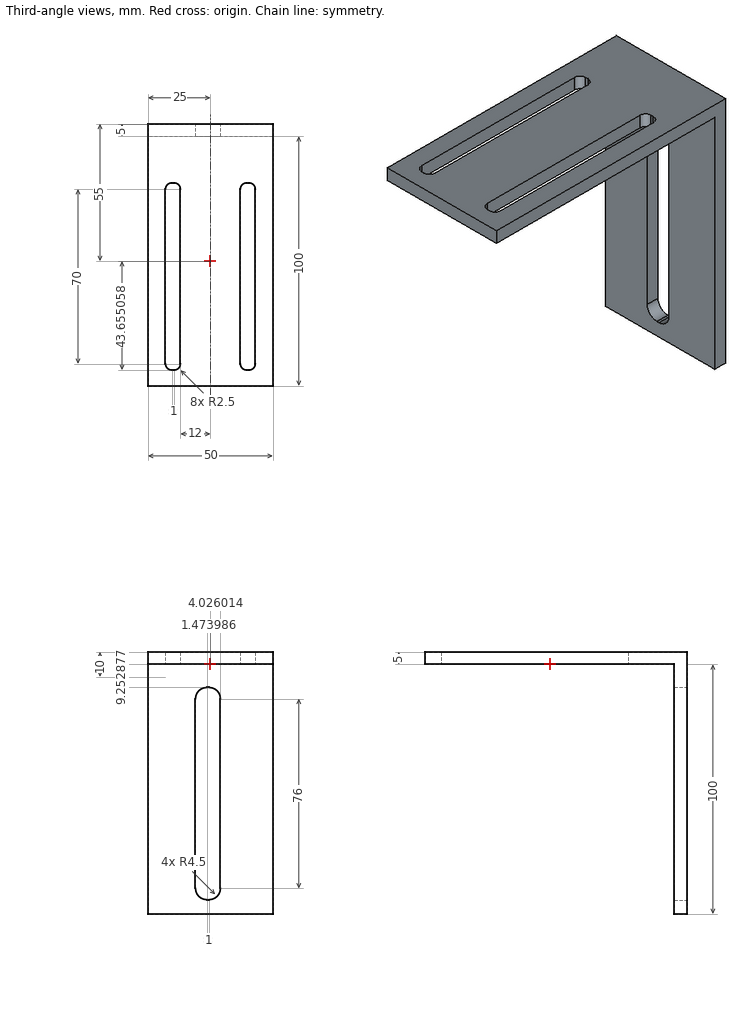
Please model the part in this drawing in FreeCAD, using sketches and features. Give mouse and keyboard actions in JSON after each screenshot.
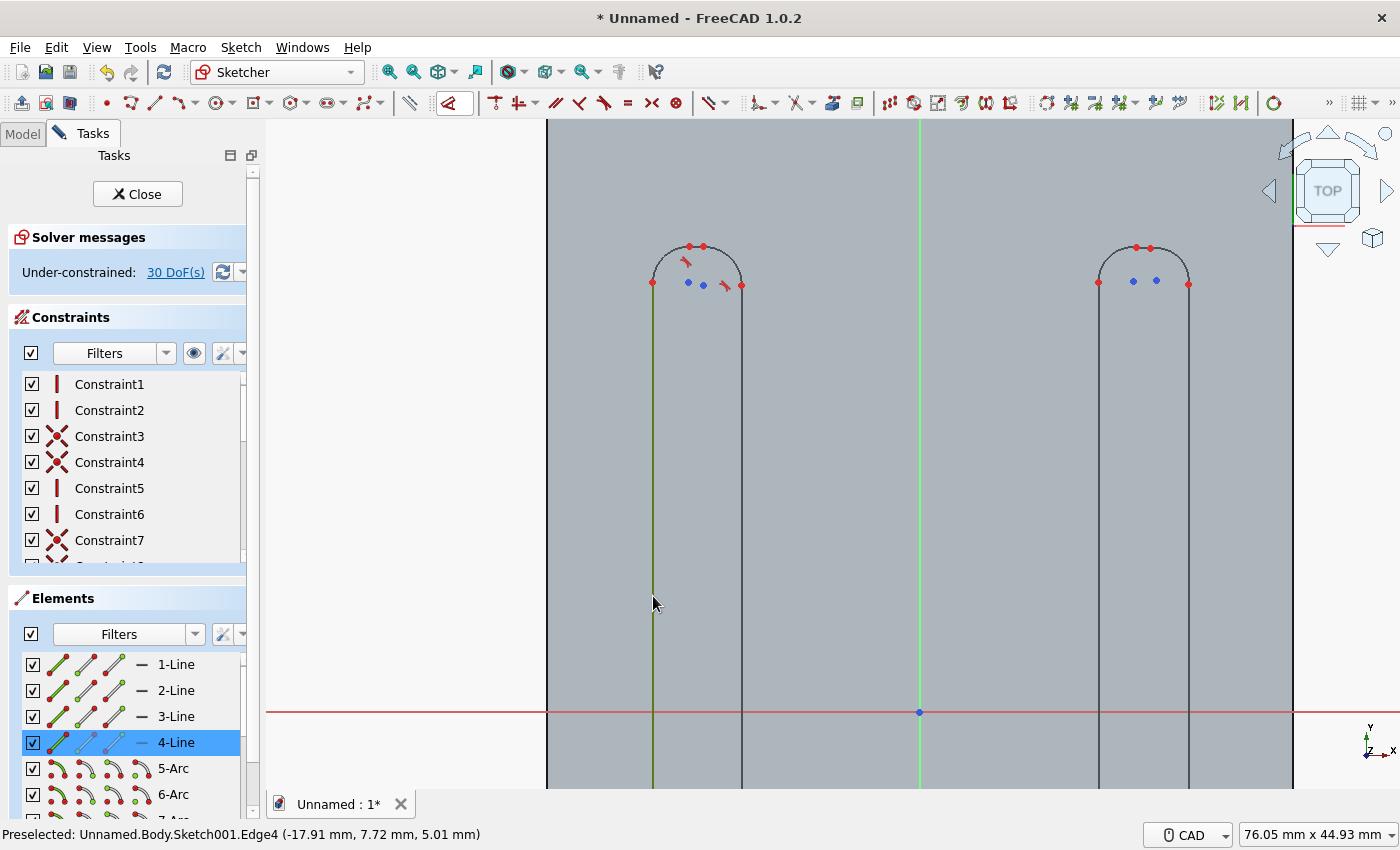
{"action": "left_click", "coordinate": [673, 251]}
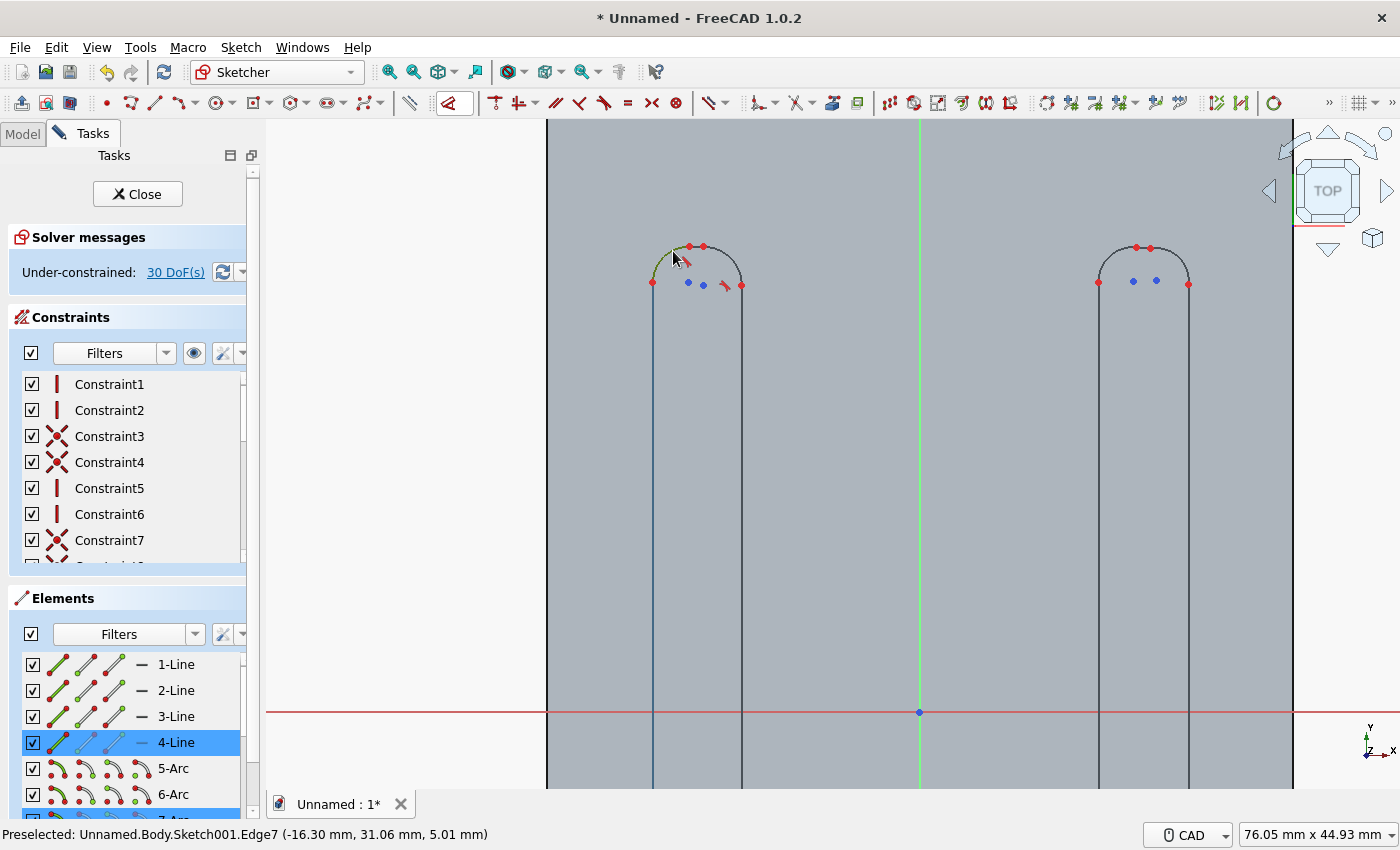
{"action": "key", "text": "t"}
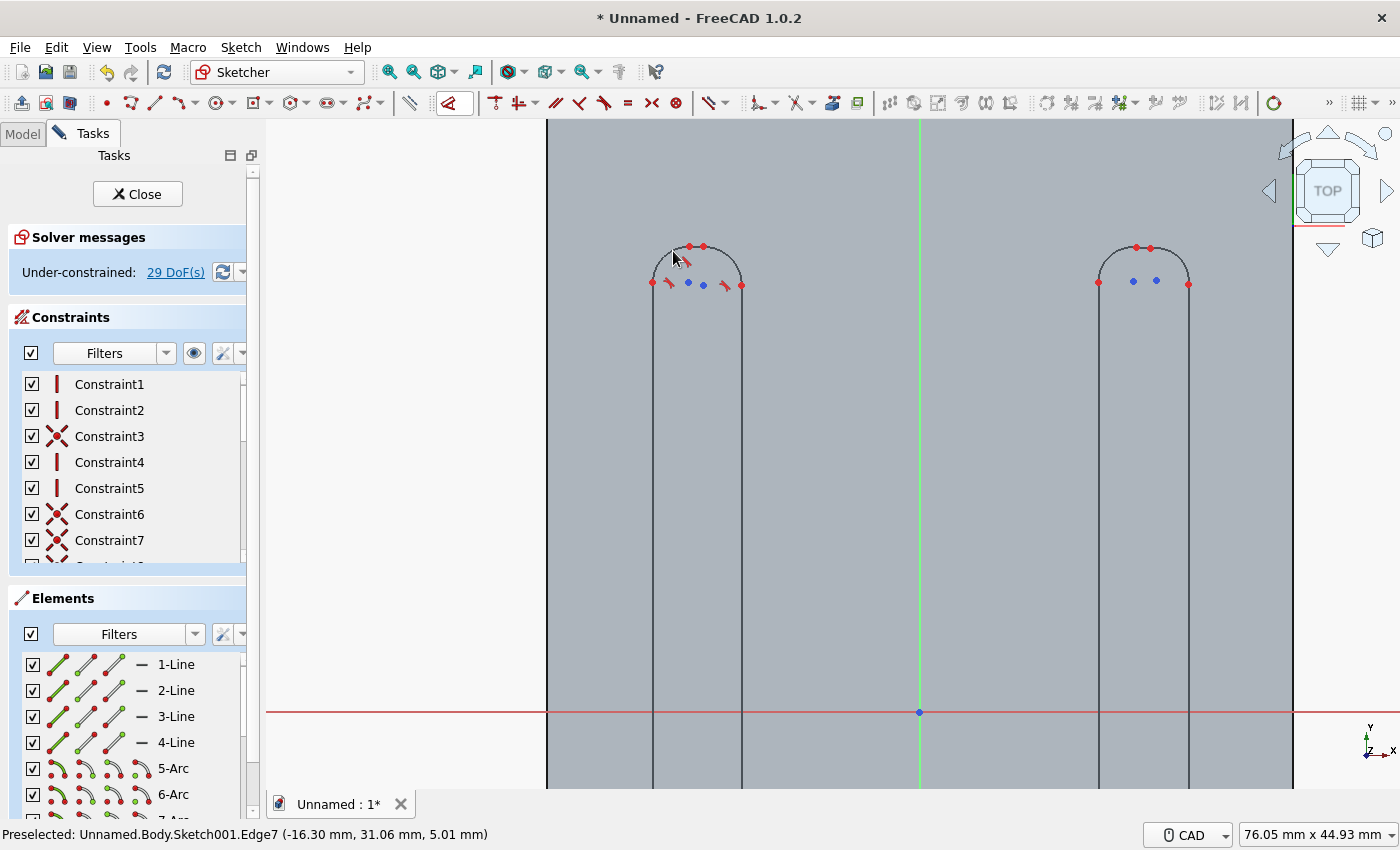
{"action": "left_click", "coordinate": [653, 596]}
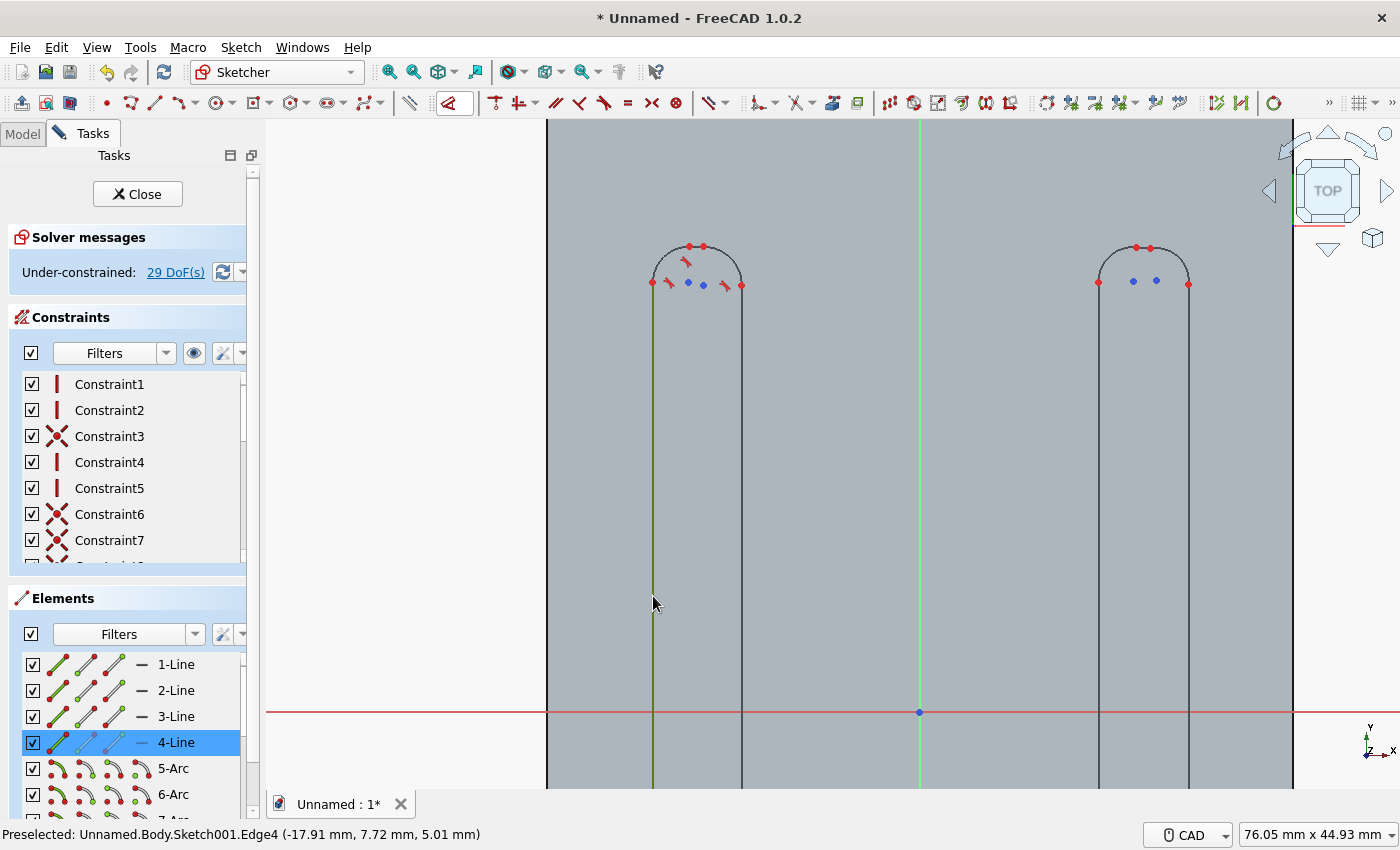
{"action": "scroll", "coordinate": [674, 250], "scroll_direction": "down", "scroll_amount": 5}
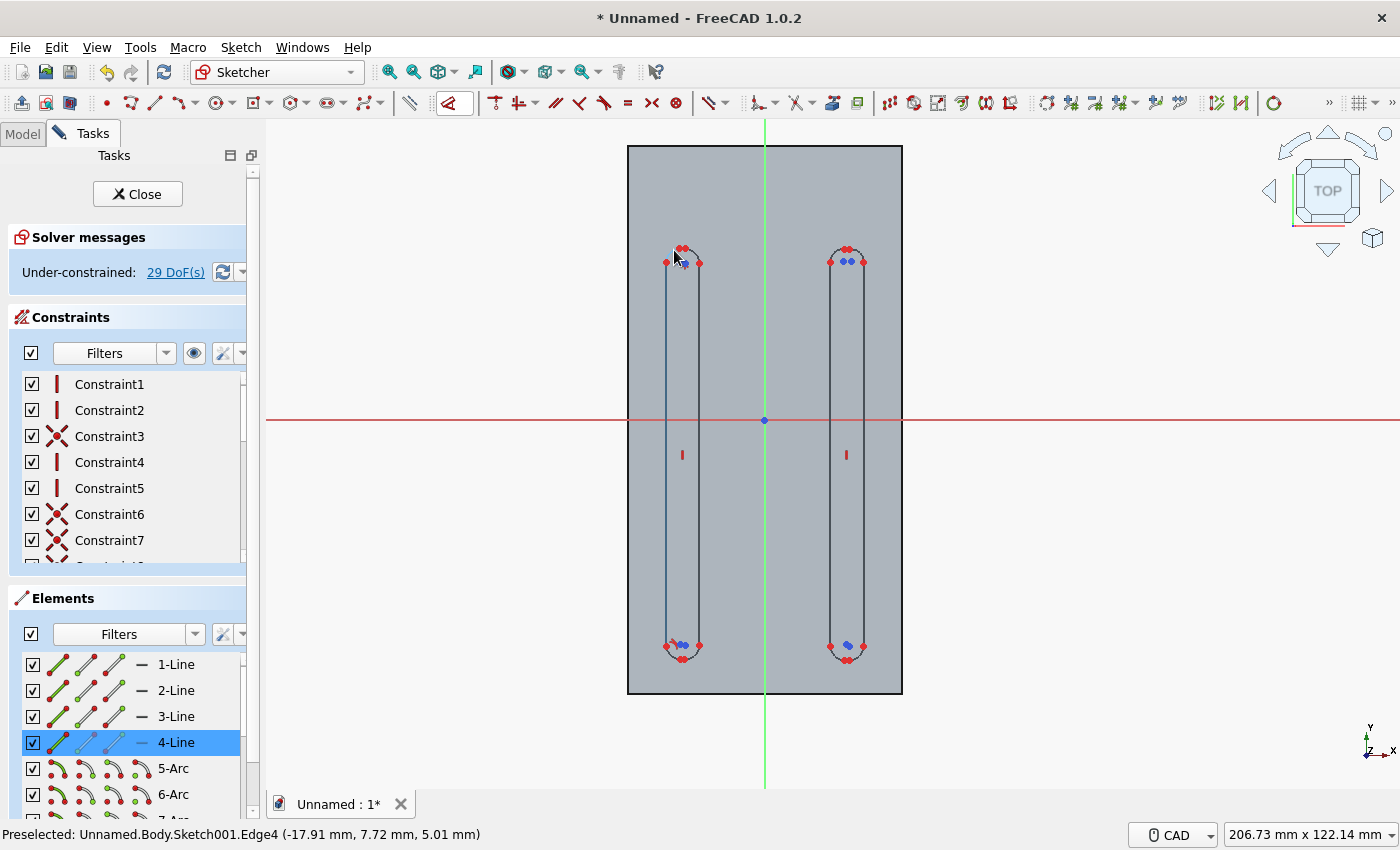
{"action": "scroll", "coordinate": [669, 653], "scroll_direction": "up", "scroll_amount": 5}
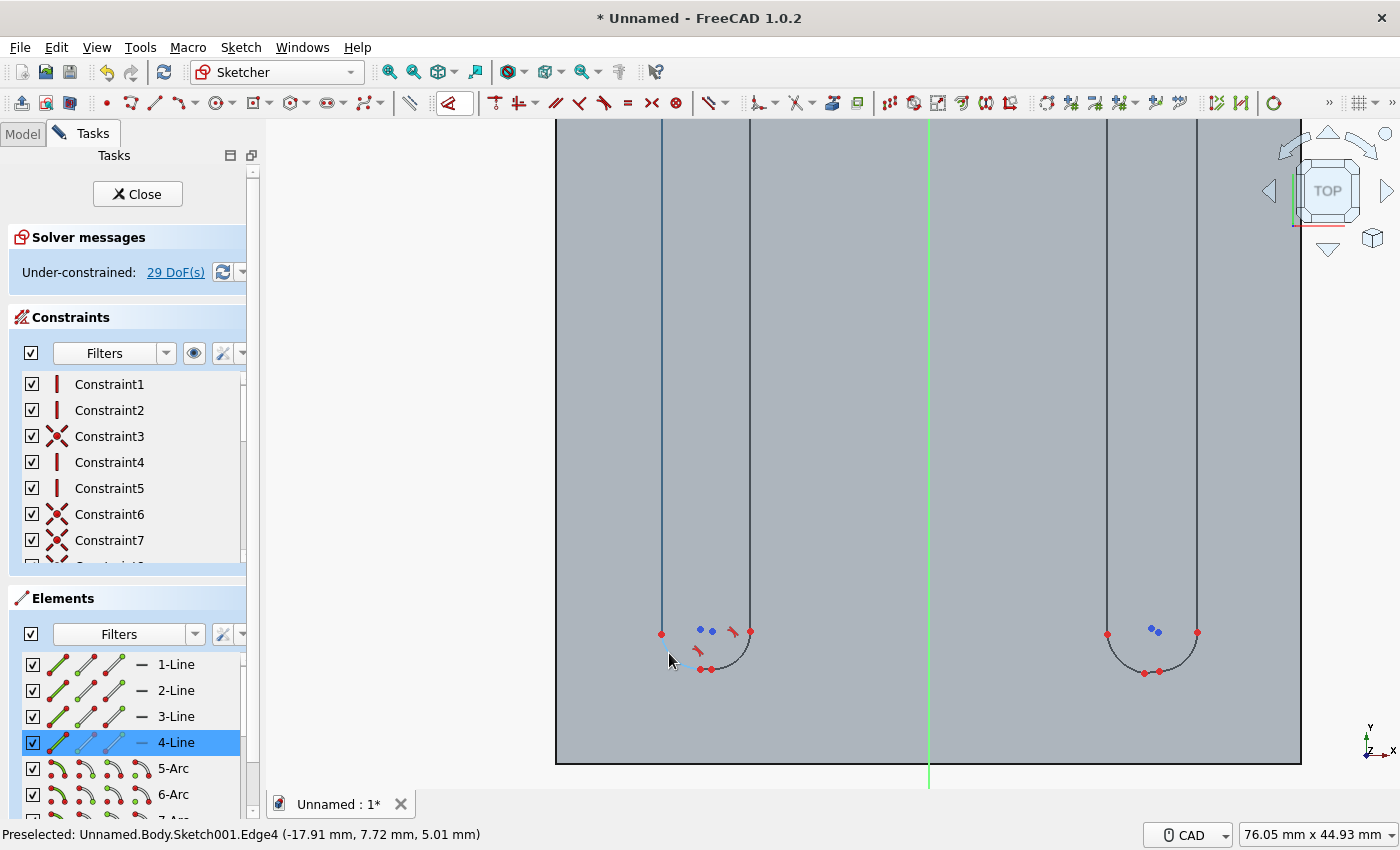
{"action": "left_click", "coordinate": [667, 651]}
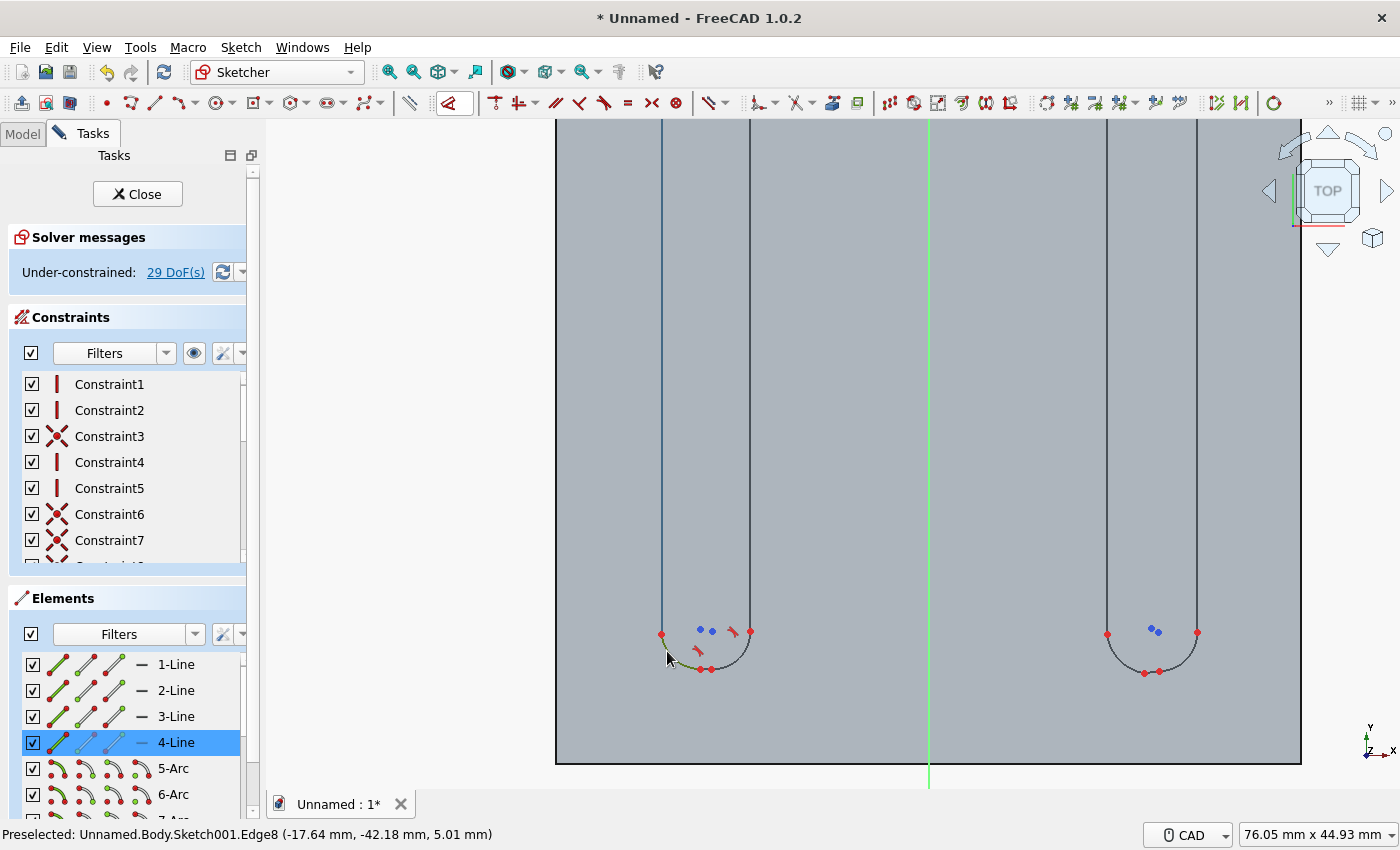
{"action": "left_click", "coordinate": [604, 104]}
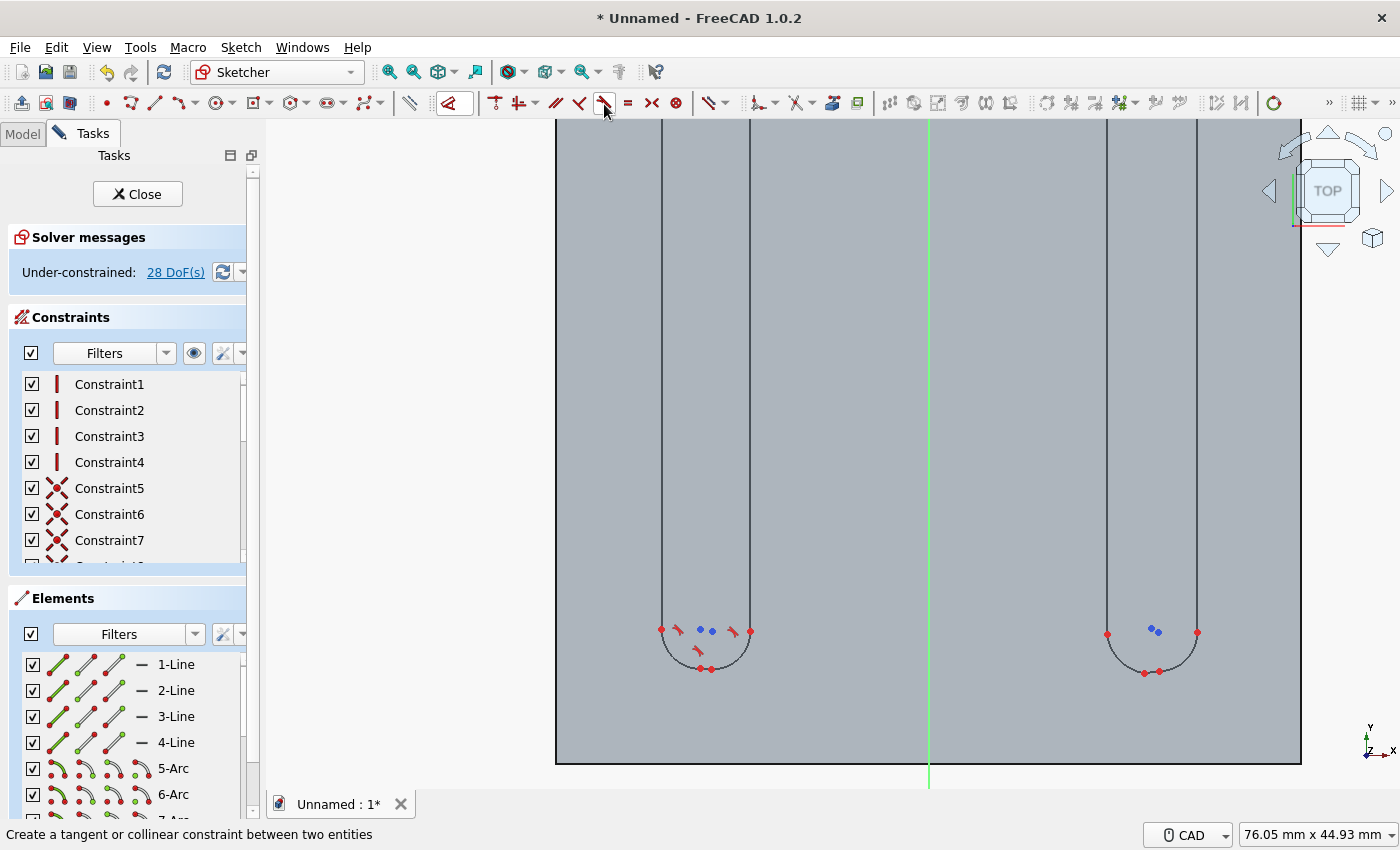
{"action": "scroll", "coordinate": [1152, 672], "scroll_direction": "up", "scroll_amount": 4}